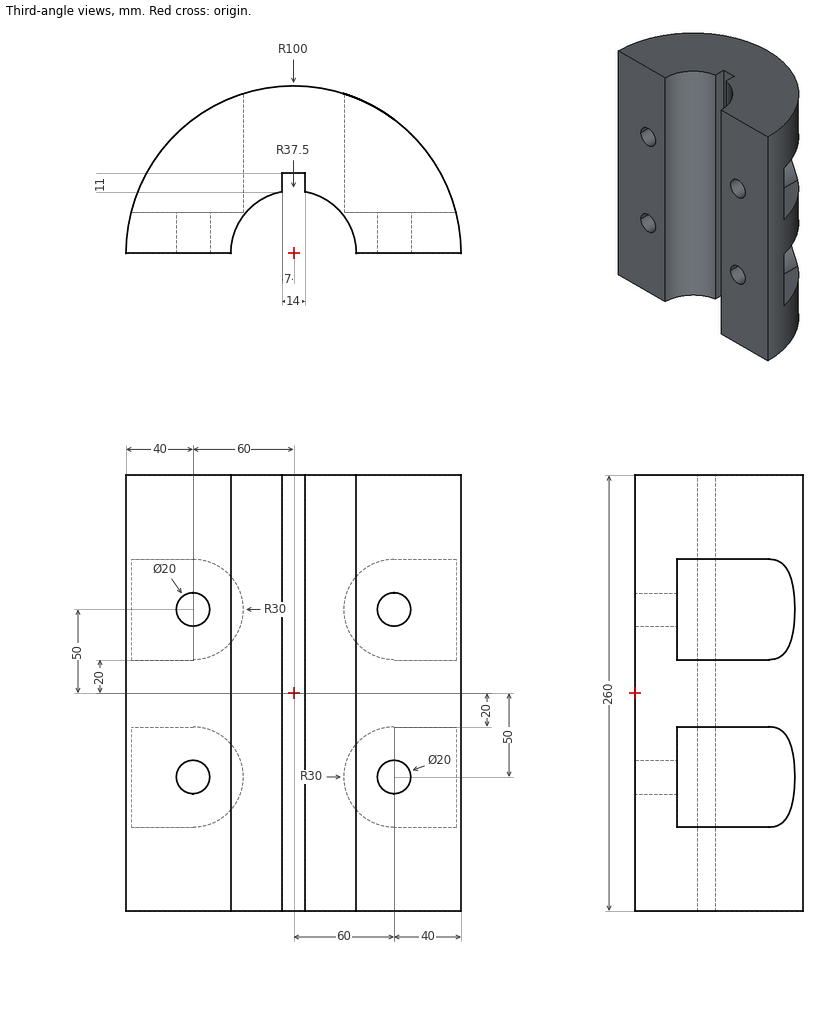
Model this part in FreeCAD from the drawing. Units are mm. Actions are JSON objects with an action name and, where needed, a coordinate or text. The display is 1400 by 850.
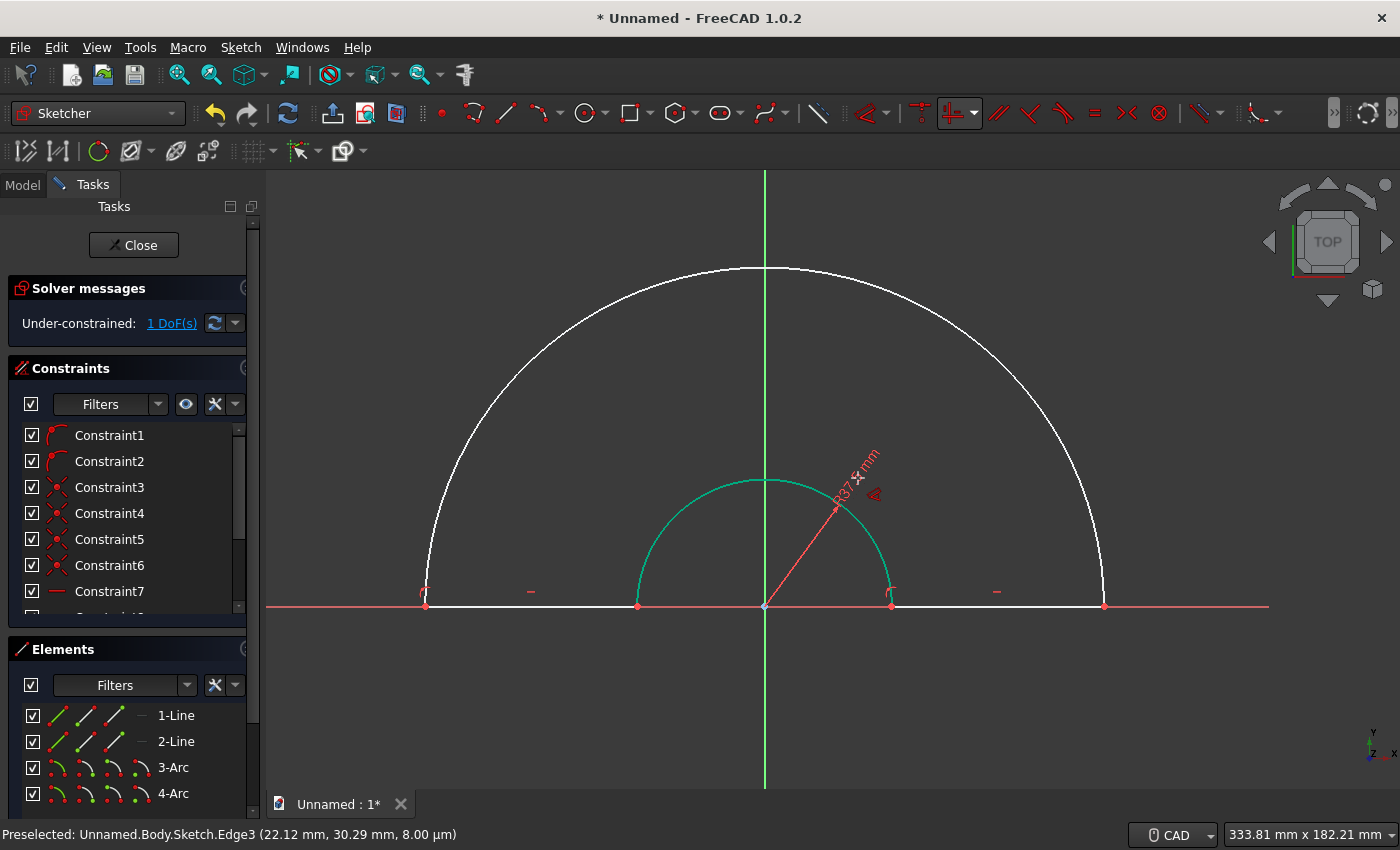
{"action": "left_click", "coordinate": [964, 332]}
{"action": "left_click", "coordinate": [983, 306]}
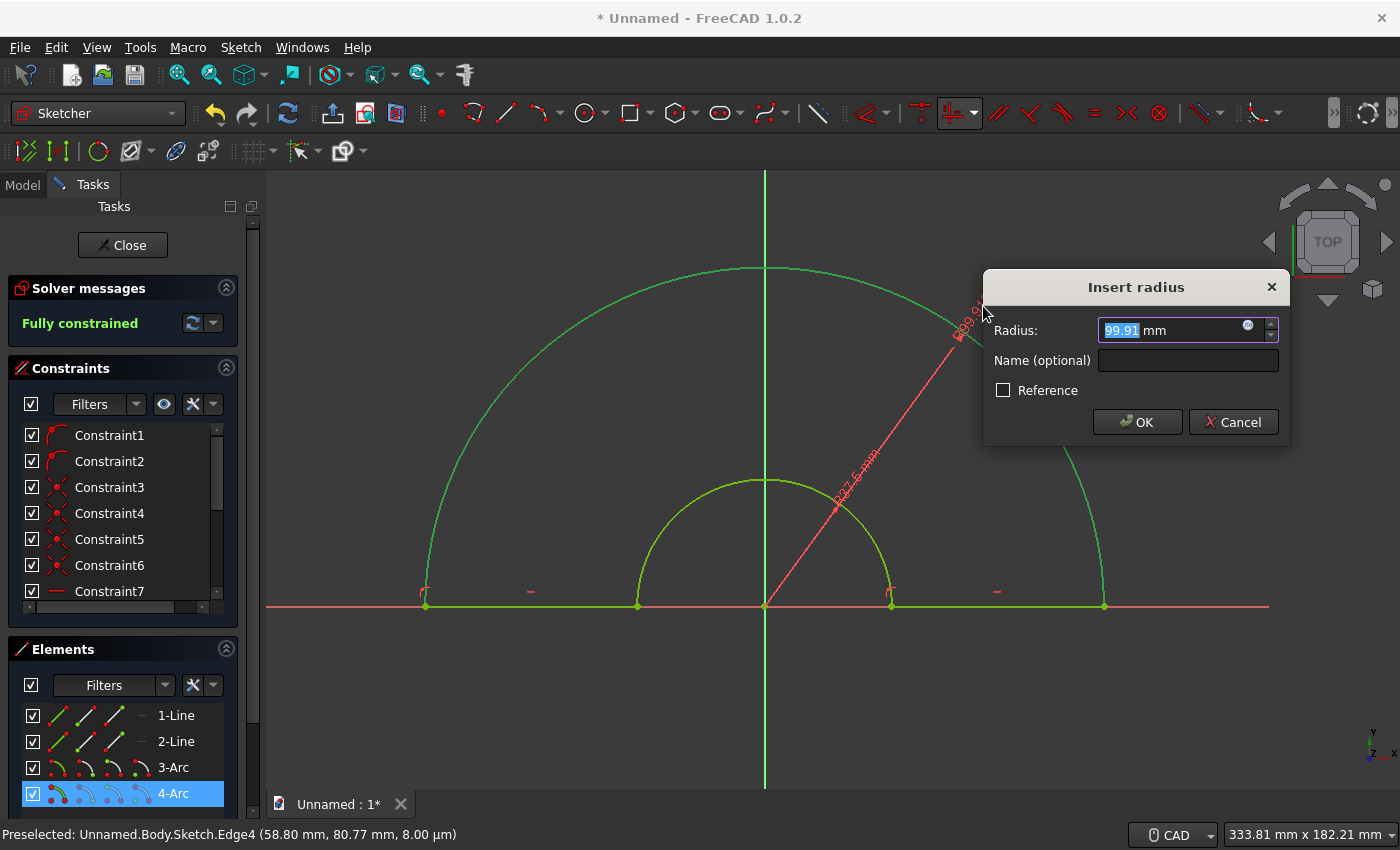
{"action": "type", "text": "100"}
{"action": "key", "text": "Return"}
{"action": "key", "text": "Escape"}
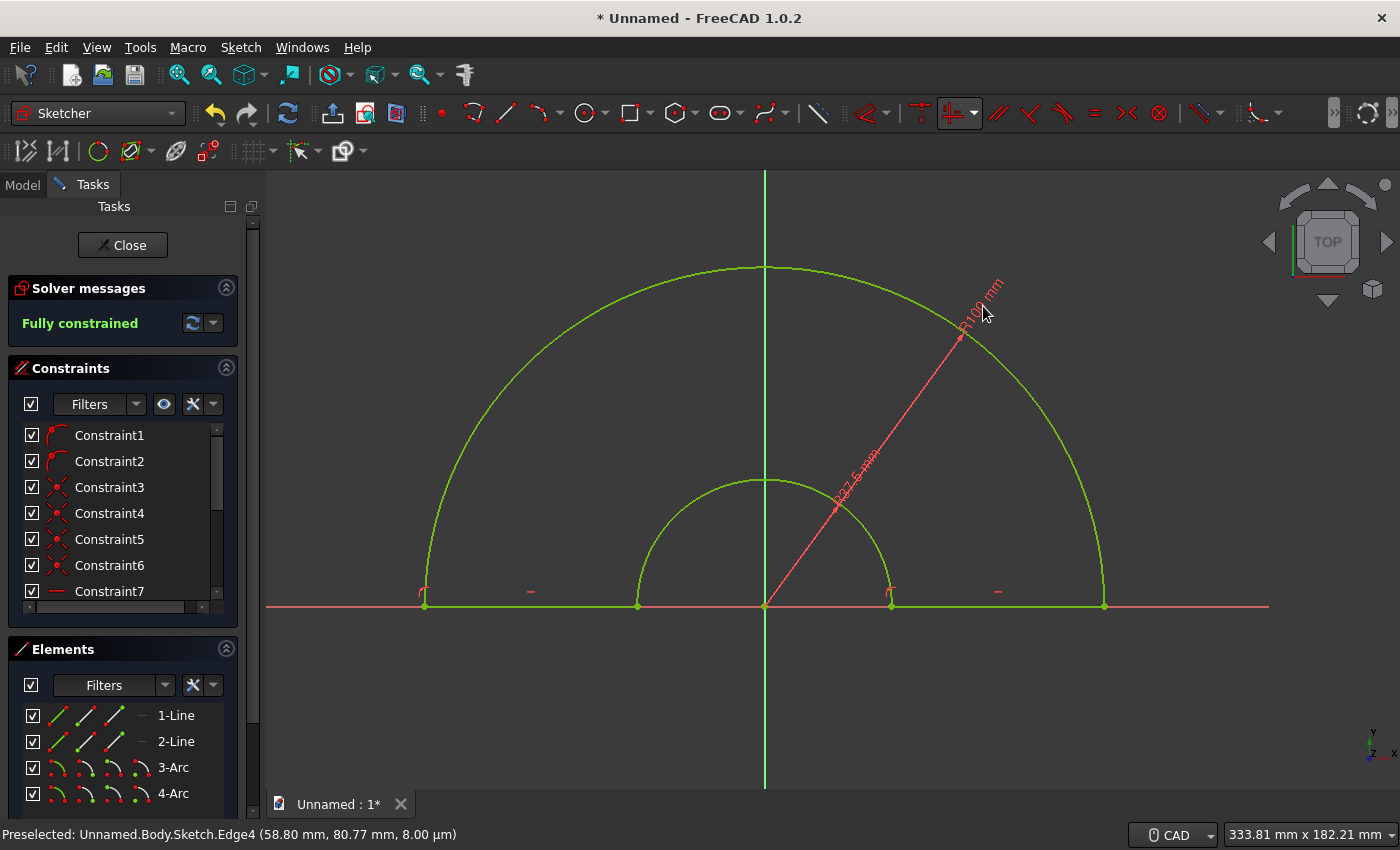
{"action": "left_click", "coordinate": [123, 245]}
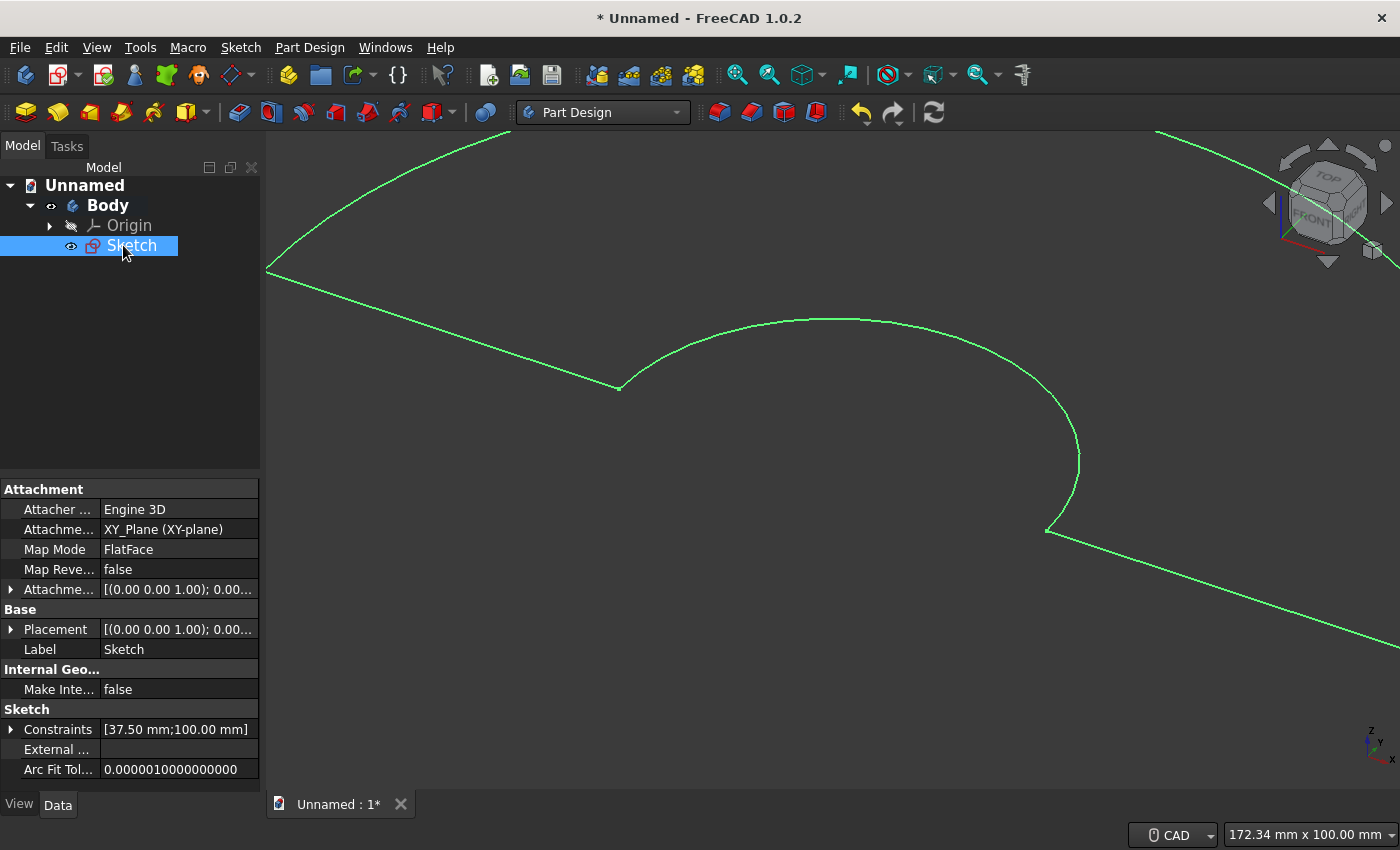
{"action": "left_click", "coordinate": [26, 112]}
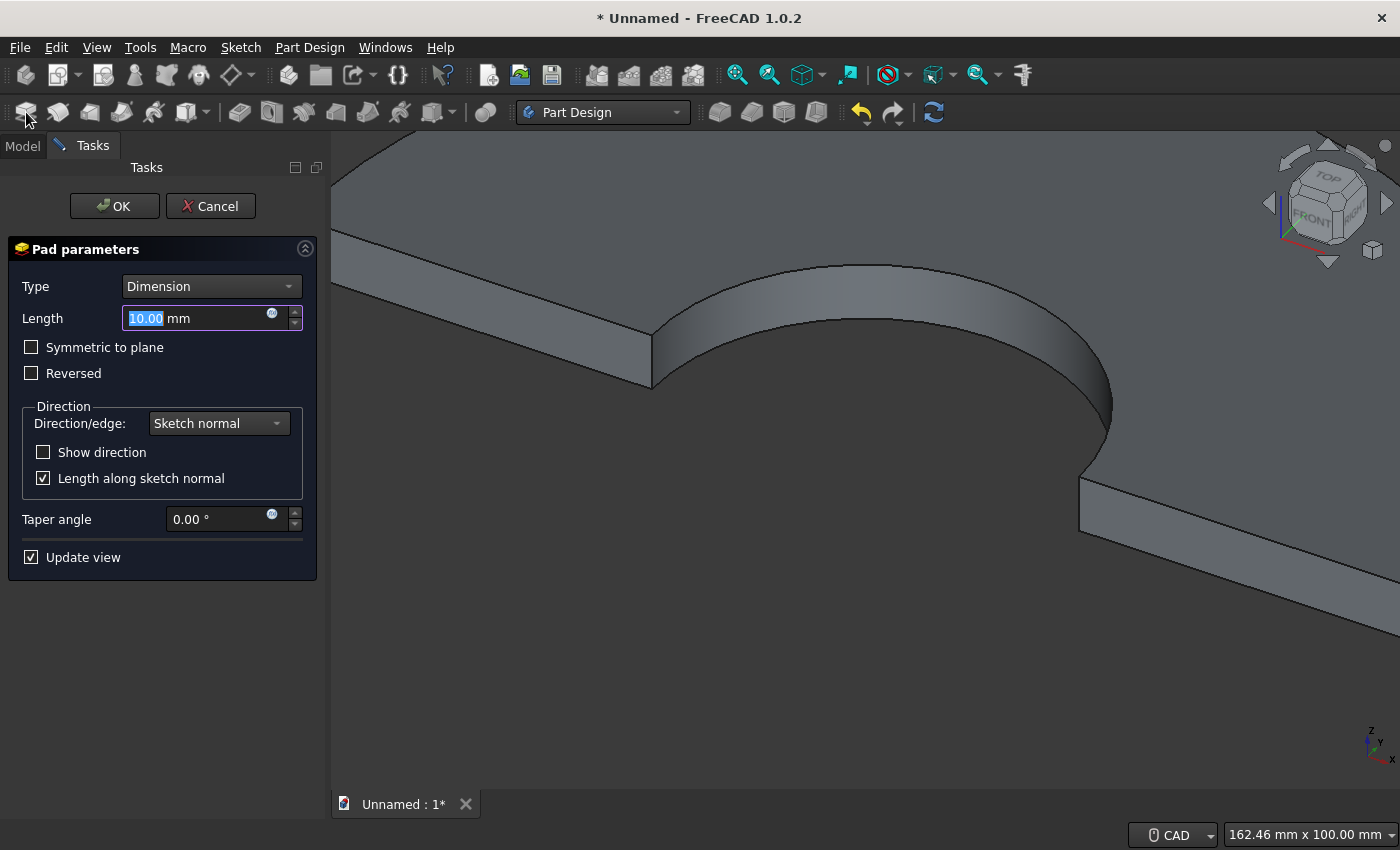
{"action": "type", "text": "260"}
{"action": "key", "text": "Tab"}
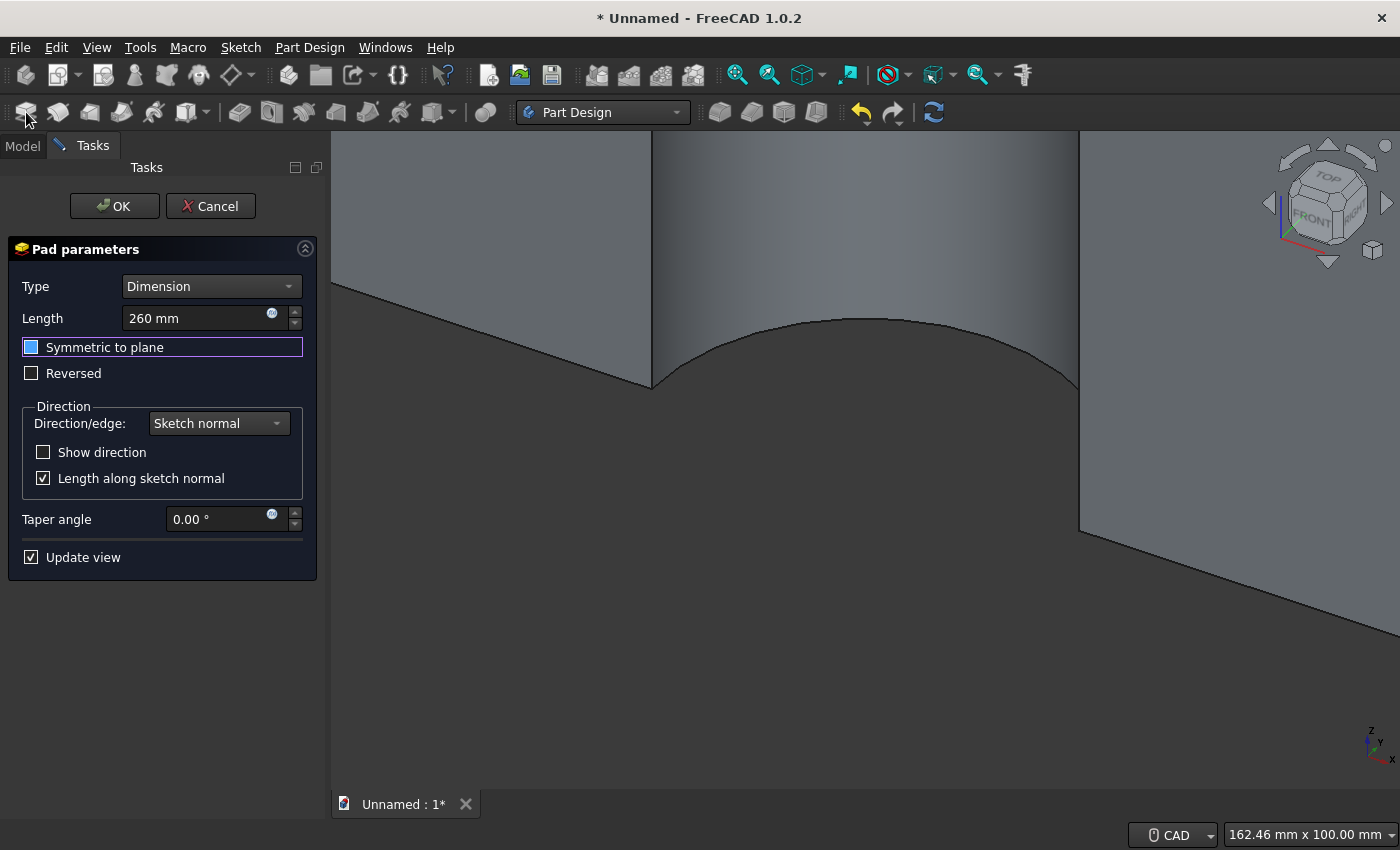
{"action": "left_click", "coordinate": [30, 347]}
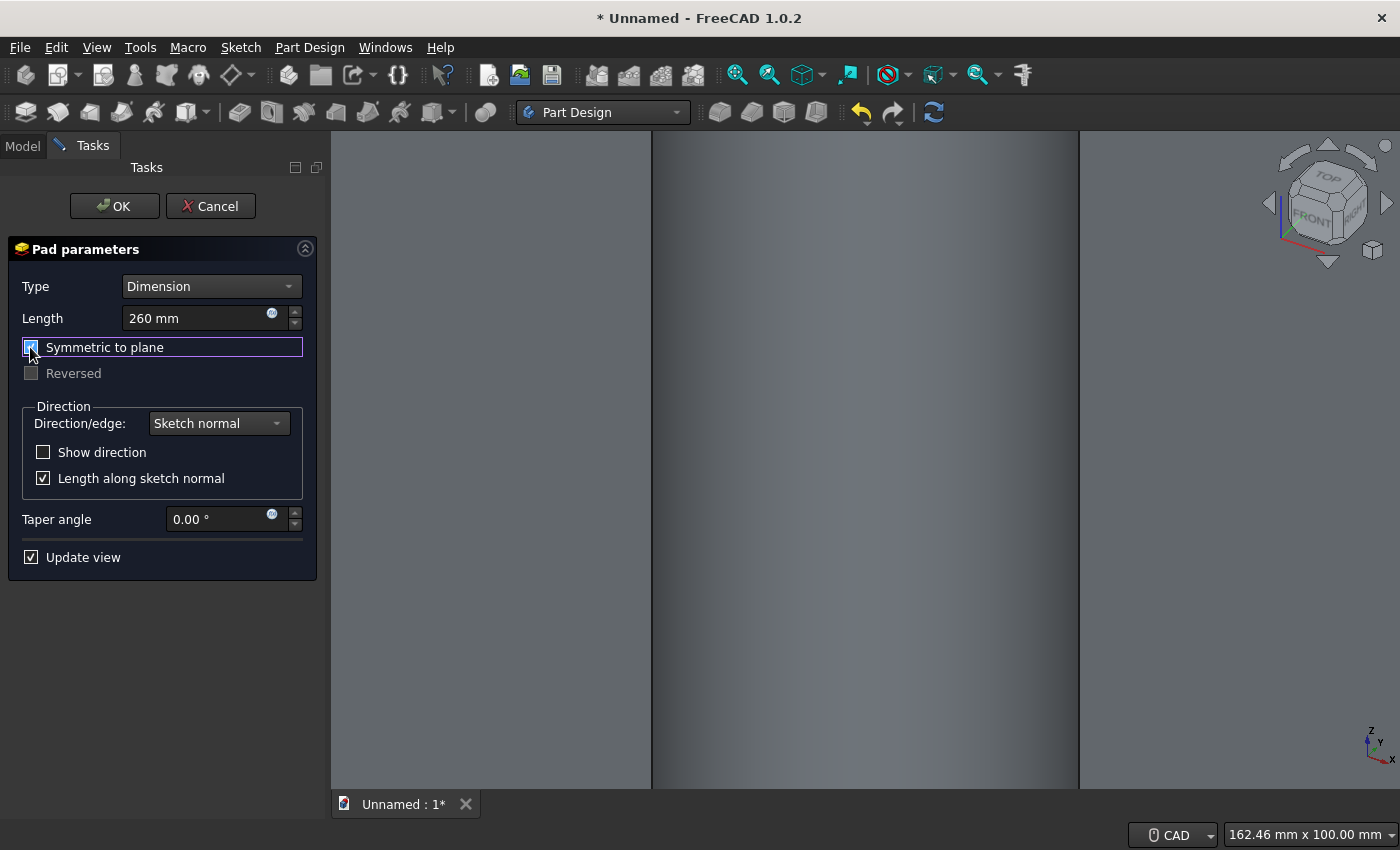
{"action": "left_click", "coordinate": [115, 206]}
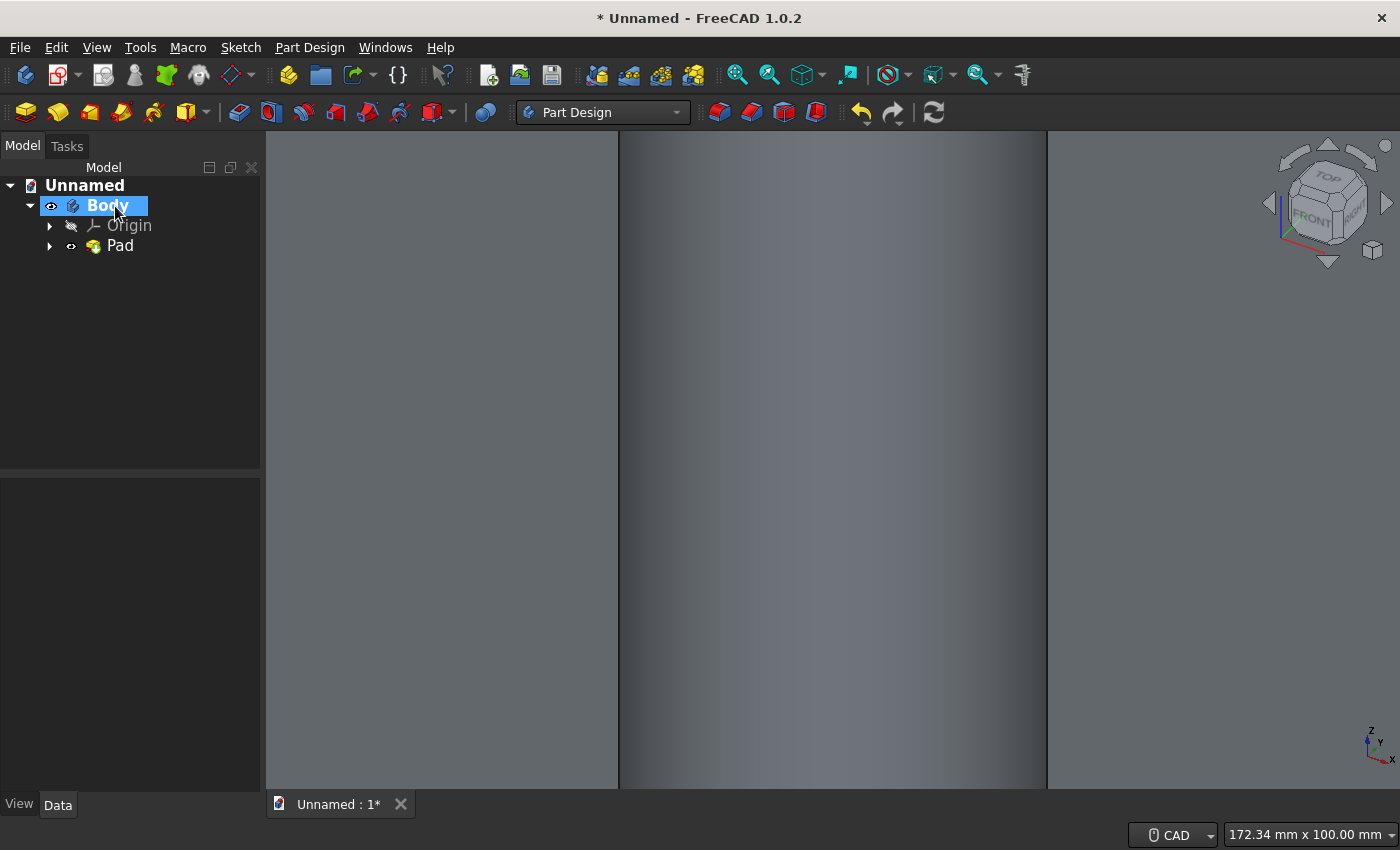
{"action": "left_click", "coordinate": [738, 76]}